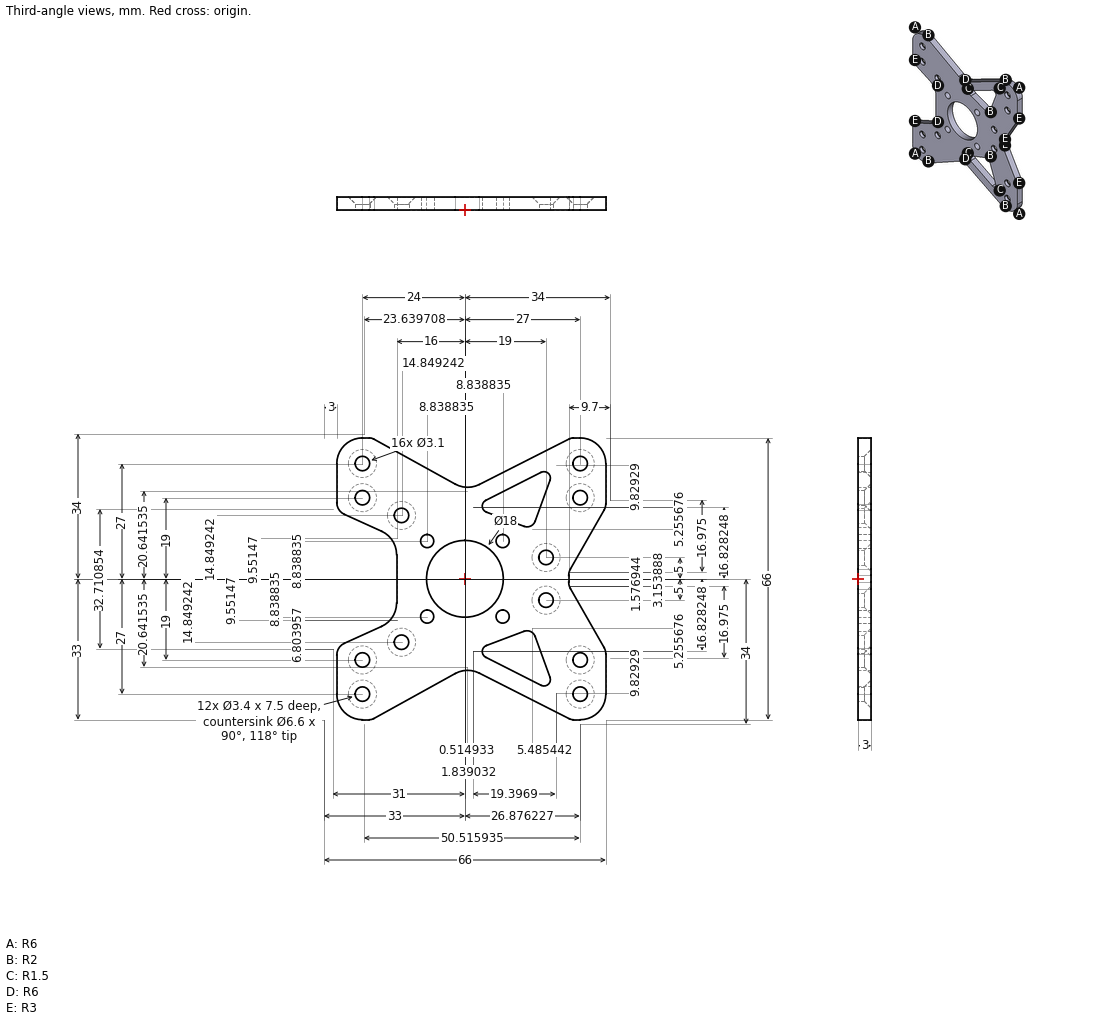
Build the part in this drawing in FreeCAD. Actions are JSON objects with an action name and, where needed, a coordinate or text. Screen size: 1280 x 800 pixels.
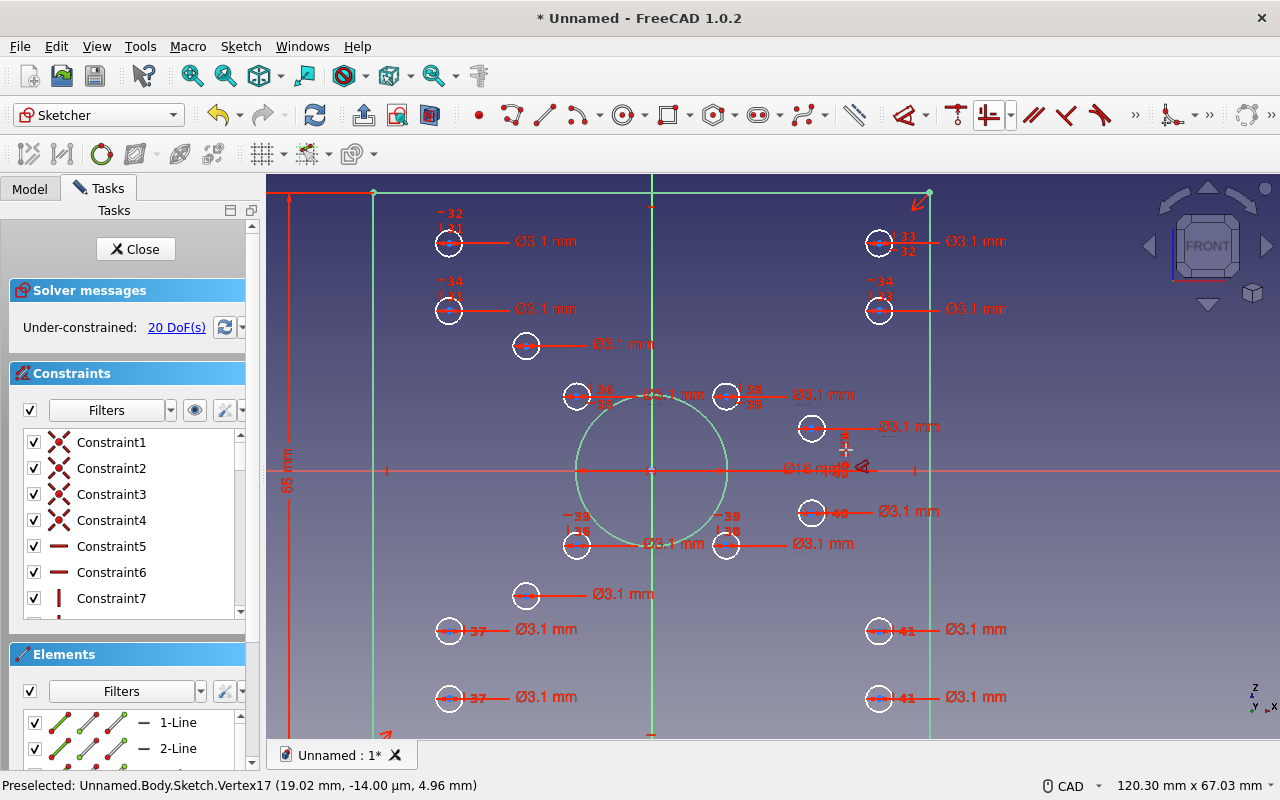
{"action": "left_click", "coordinate": [812, 513]}
{"action": "left_click", "coordinate": [846, 492]}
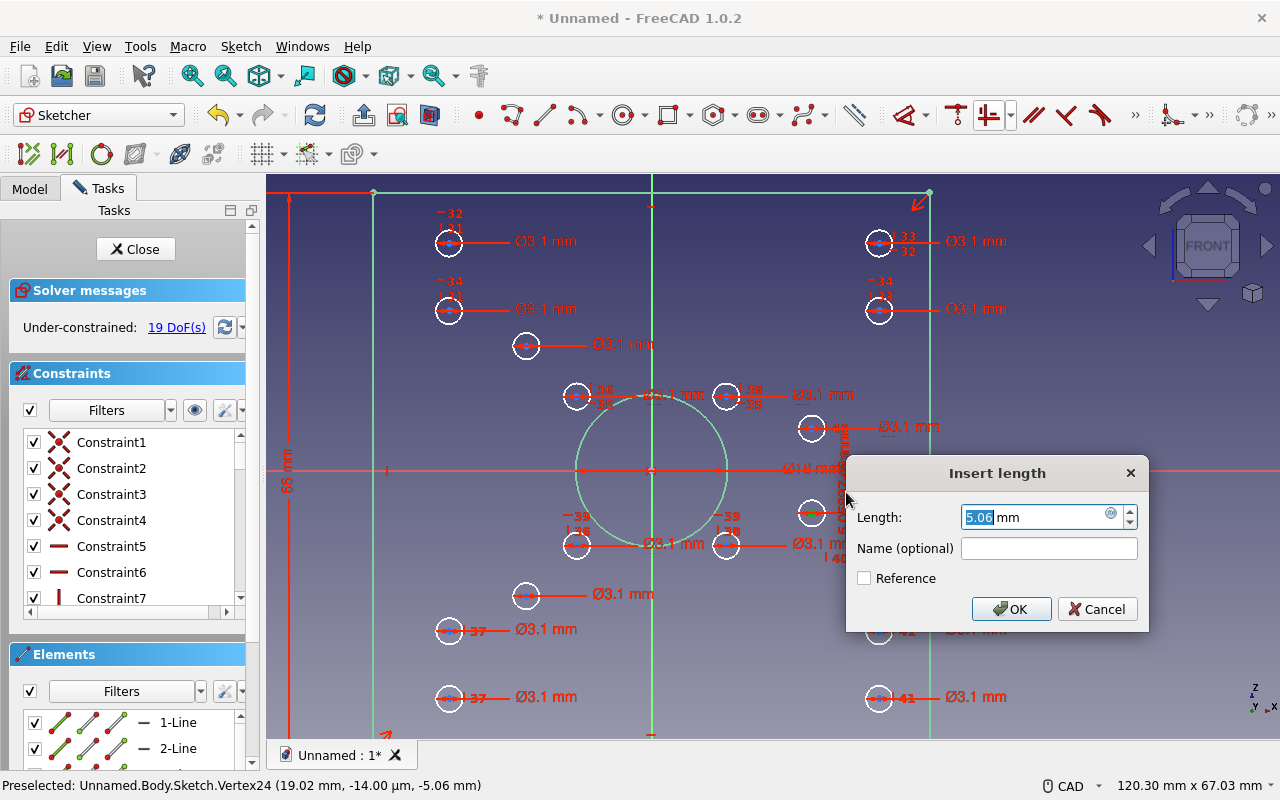
{"action": "type", "text": "5"}
{"action": "key", "text": "Return"}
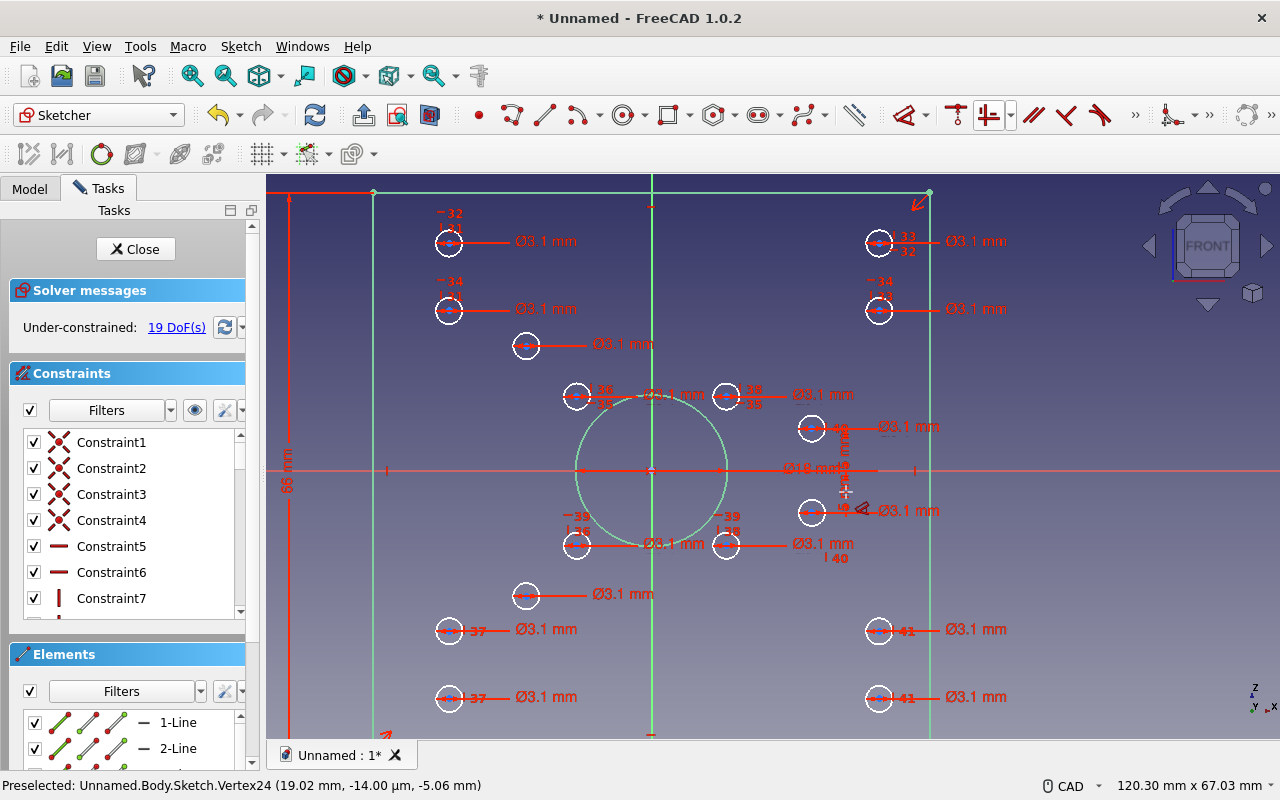
{"action": "left_click", "coordinate": [449, 243]}
{"action": "left_click", "coordinate": [550, 209]}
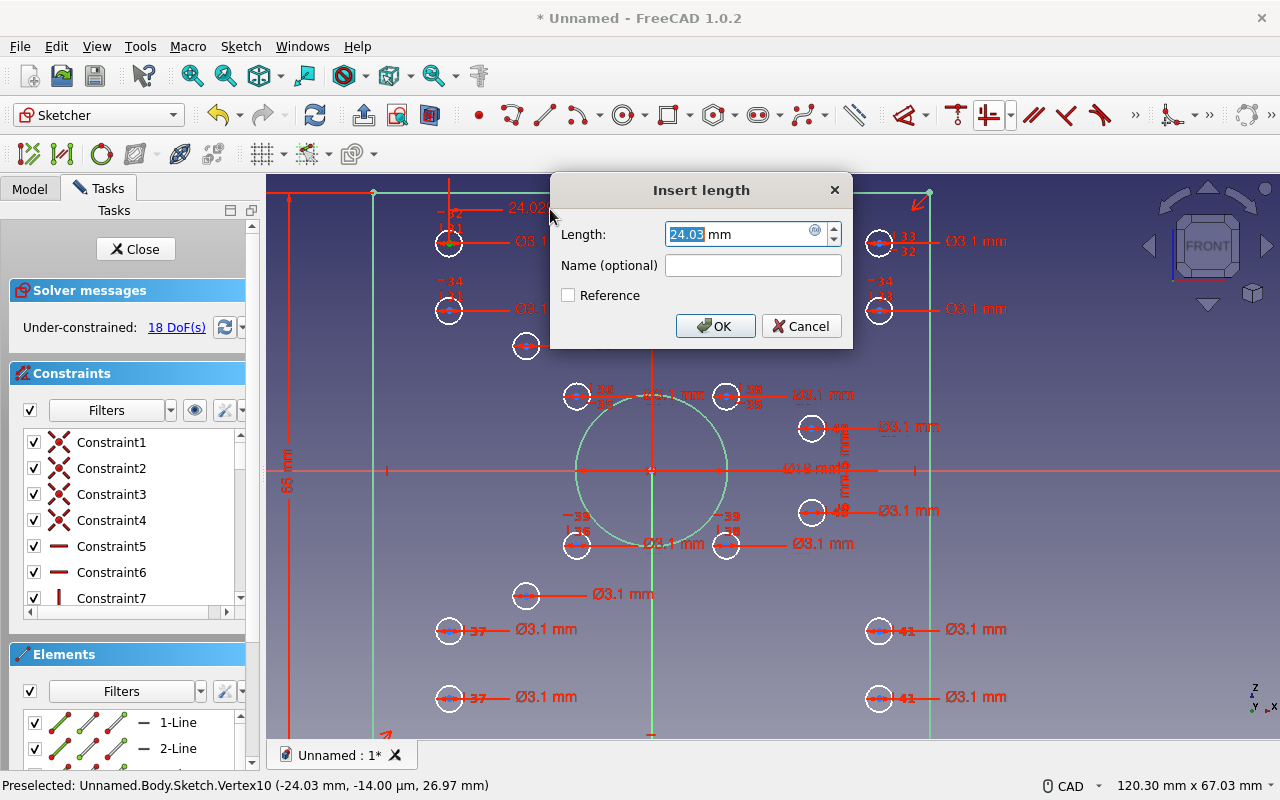
{"action": "type", "text": "24"}
{"action": "key", "text": "Return"}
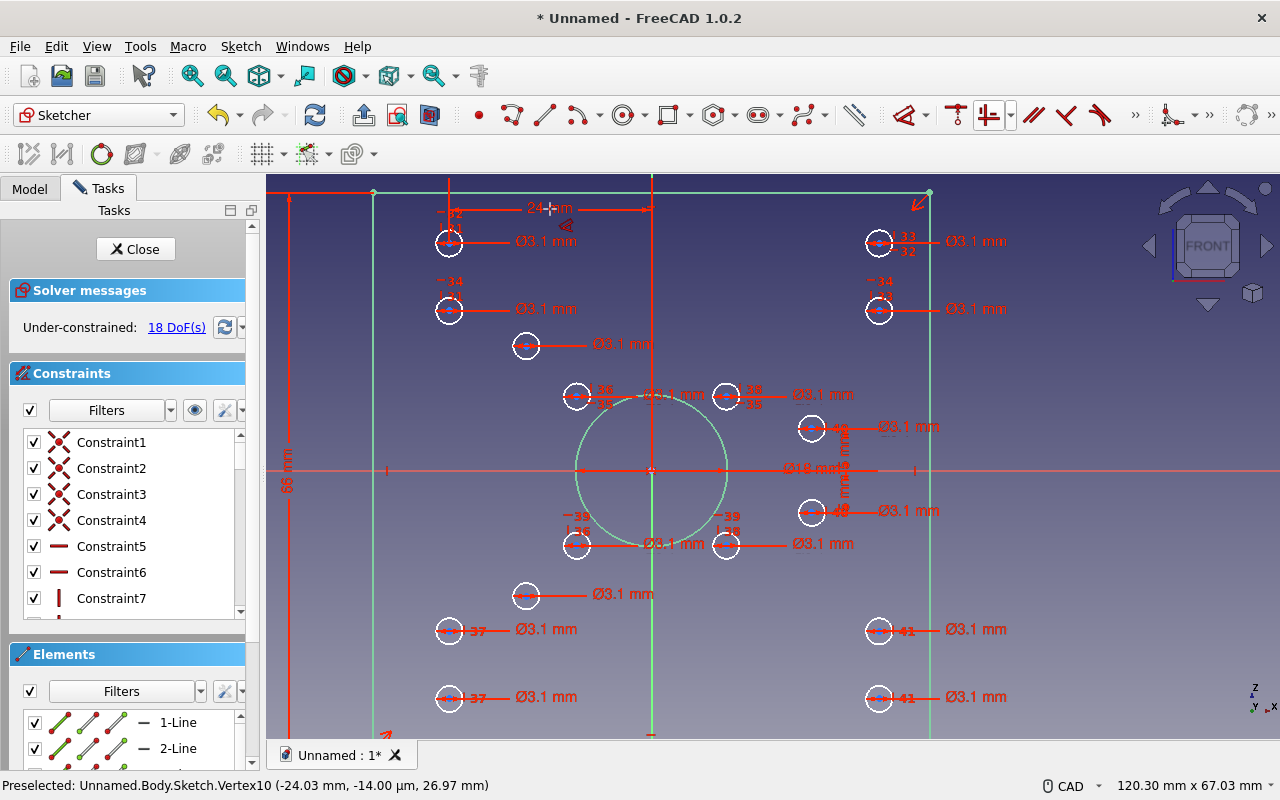
{"action": "left_click", "coordinate": [449, 243]}
{"action": "left_click", "coordinate": [415, 357]}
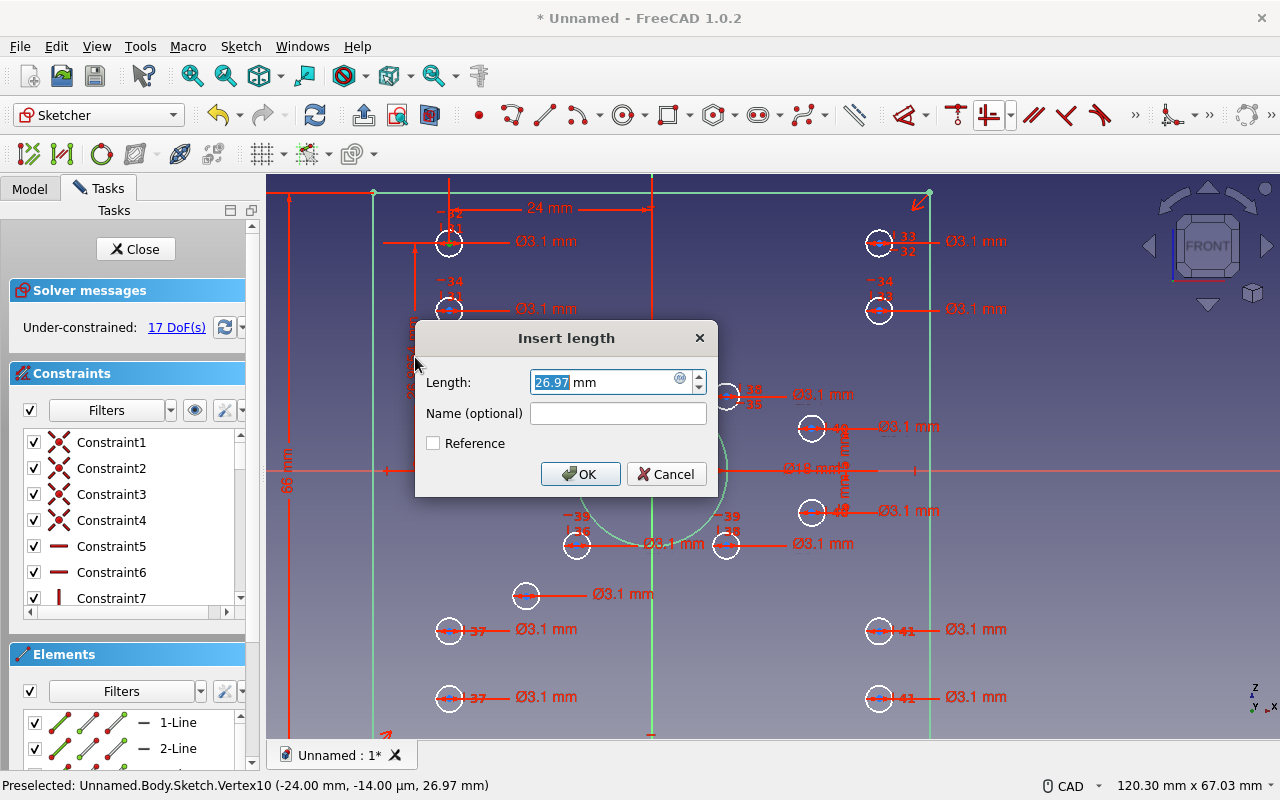
{"action": "type", "text": "27"}
{"action": "key", "text": "Return"}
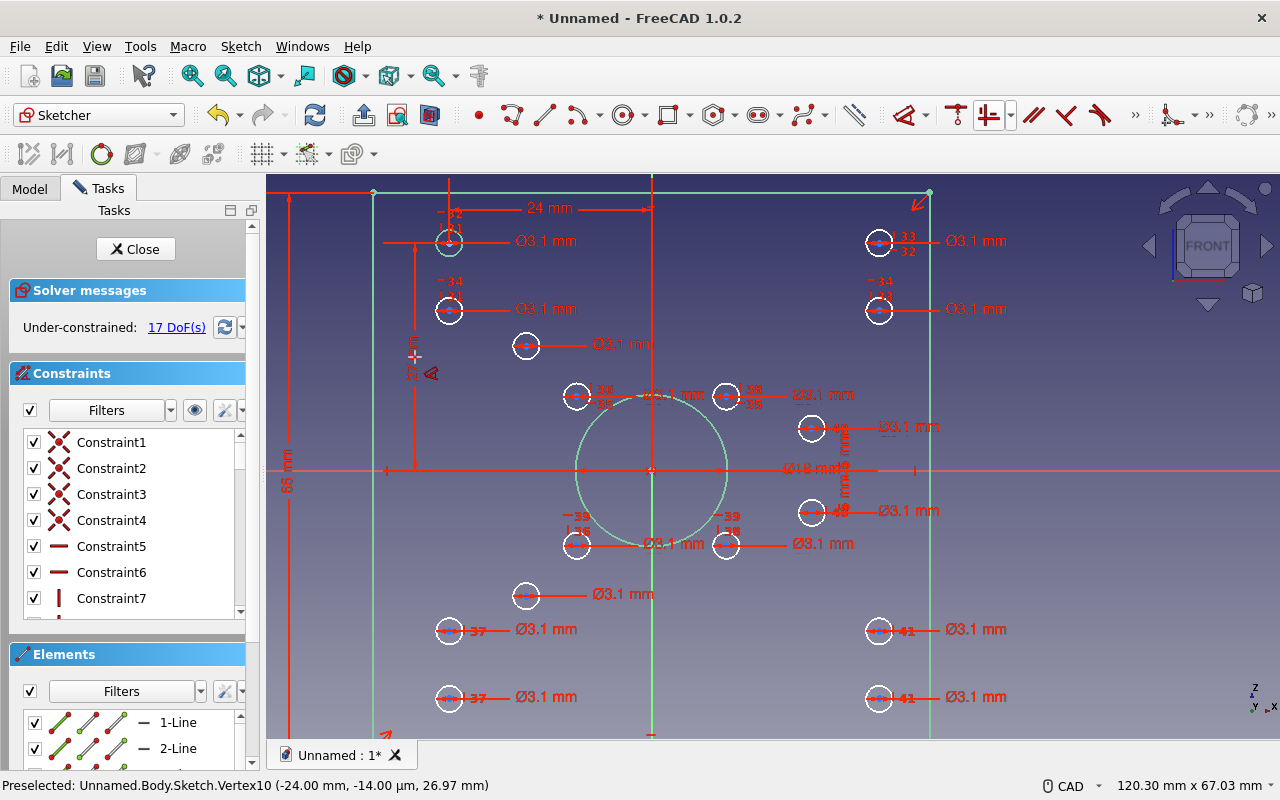
{"action": "left_click", "coordinate": [449, 311]}
{"action": "left_click", "coordinate": [415, 391]}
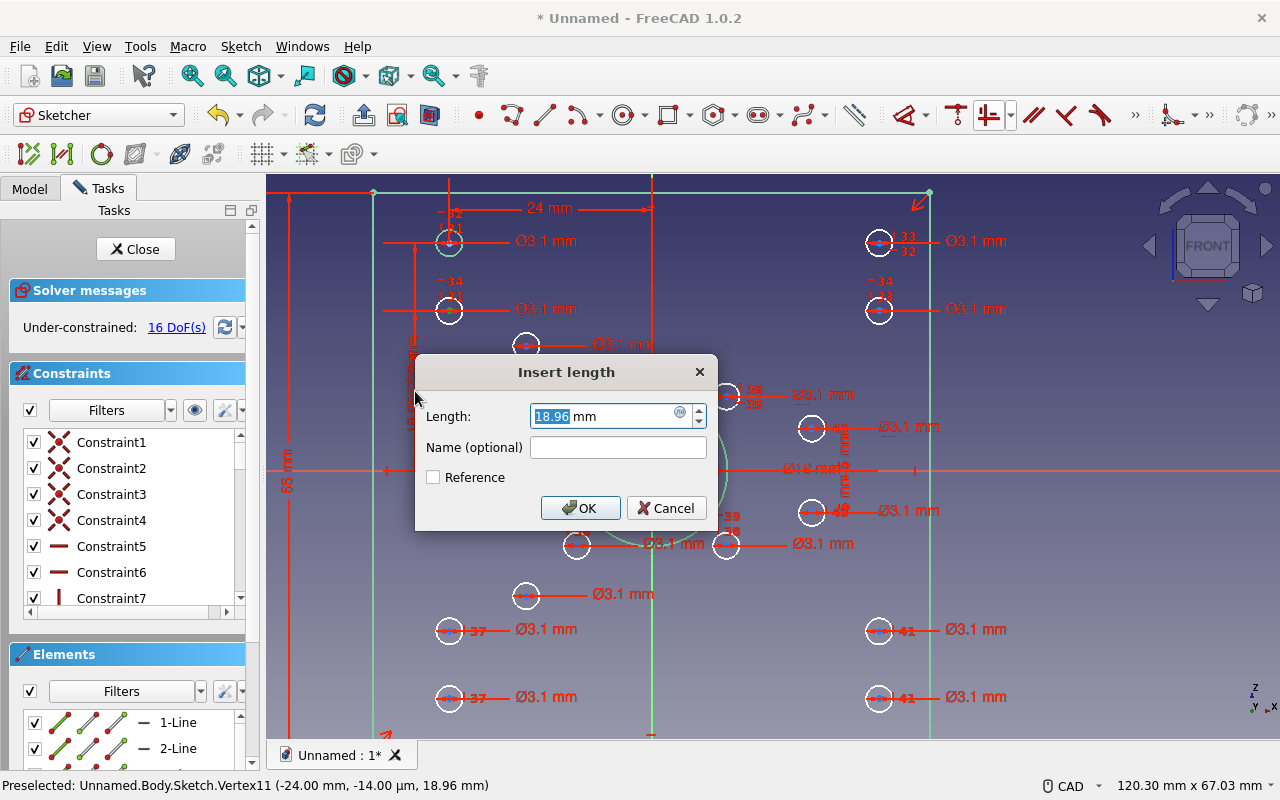
{"action": "type", "text": "19"}
{"action": "key", "text": "Return"}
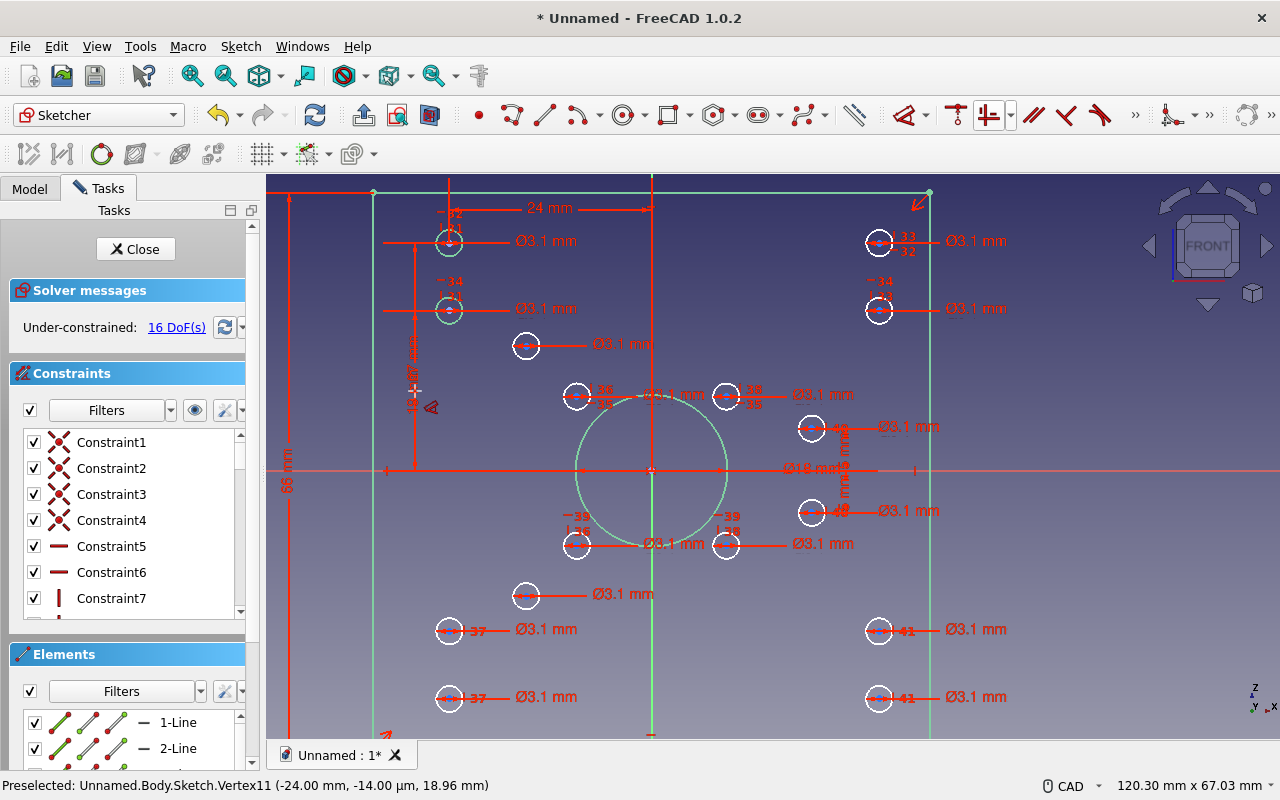
{"action": "left_click", "coordinate": [879, 243]}
{"action": "left_click", "coordinate": [766, 209]}